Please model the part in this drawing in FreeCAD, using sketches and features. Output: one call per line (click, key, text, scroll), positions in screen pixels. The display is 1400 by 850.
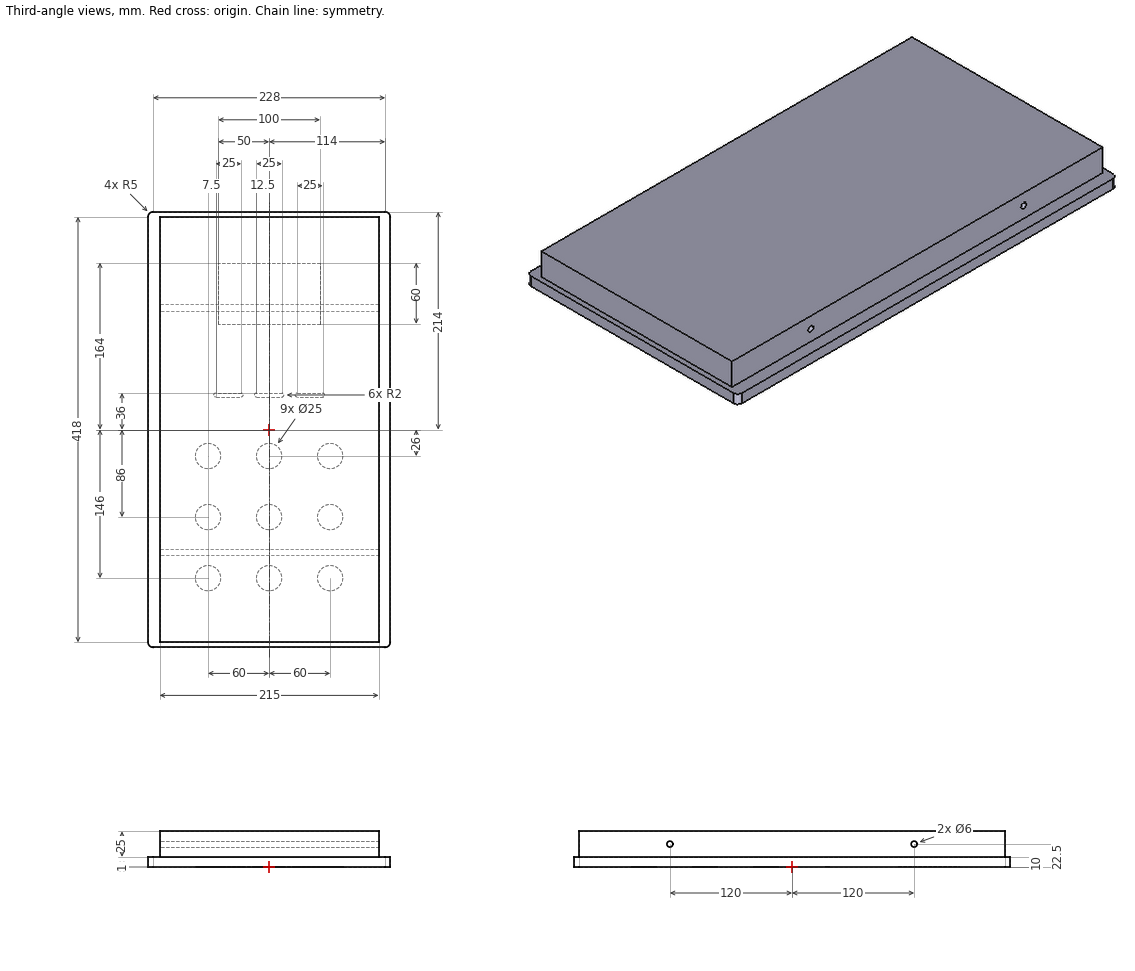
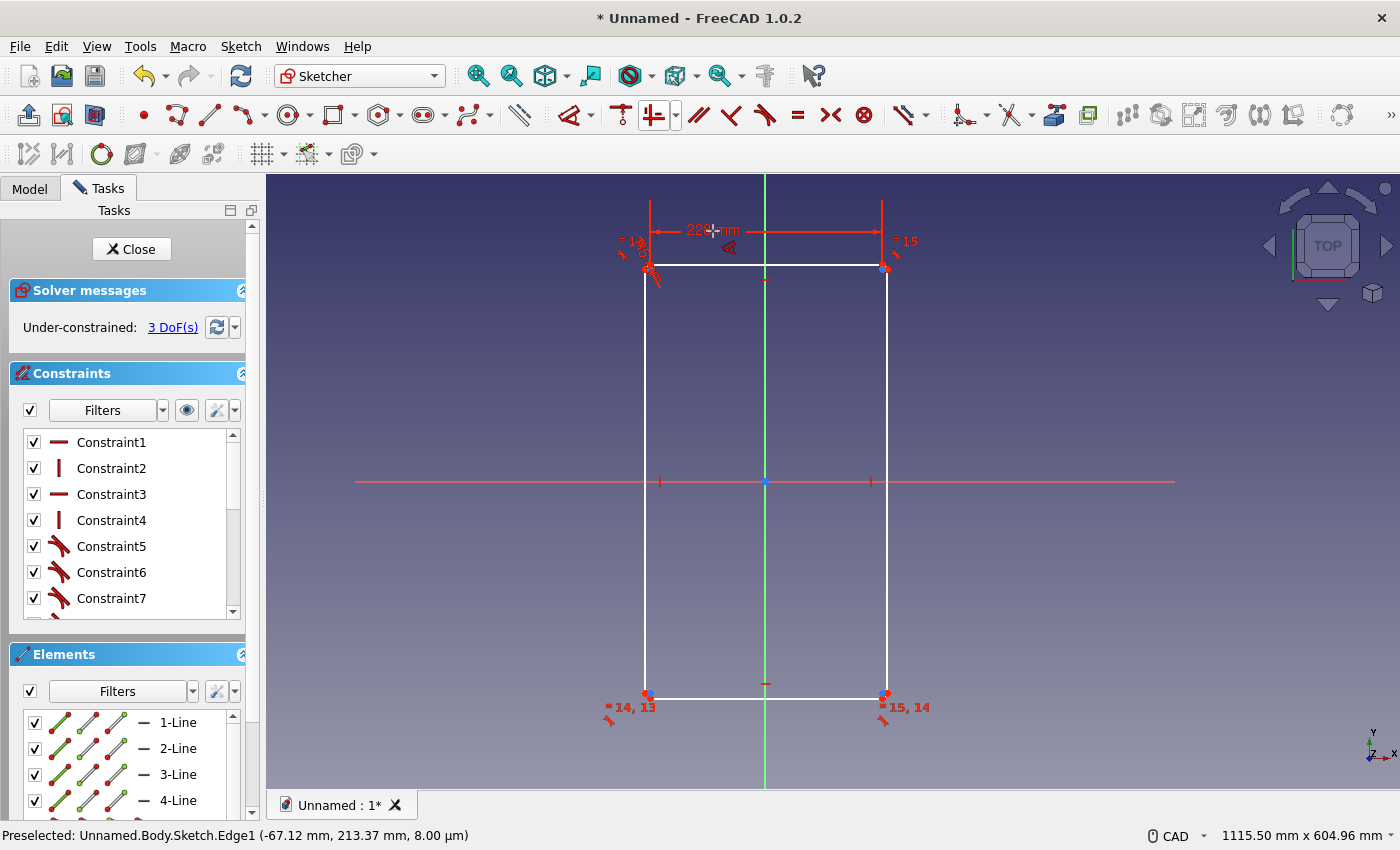
click(645, 397)
click(611, 384)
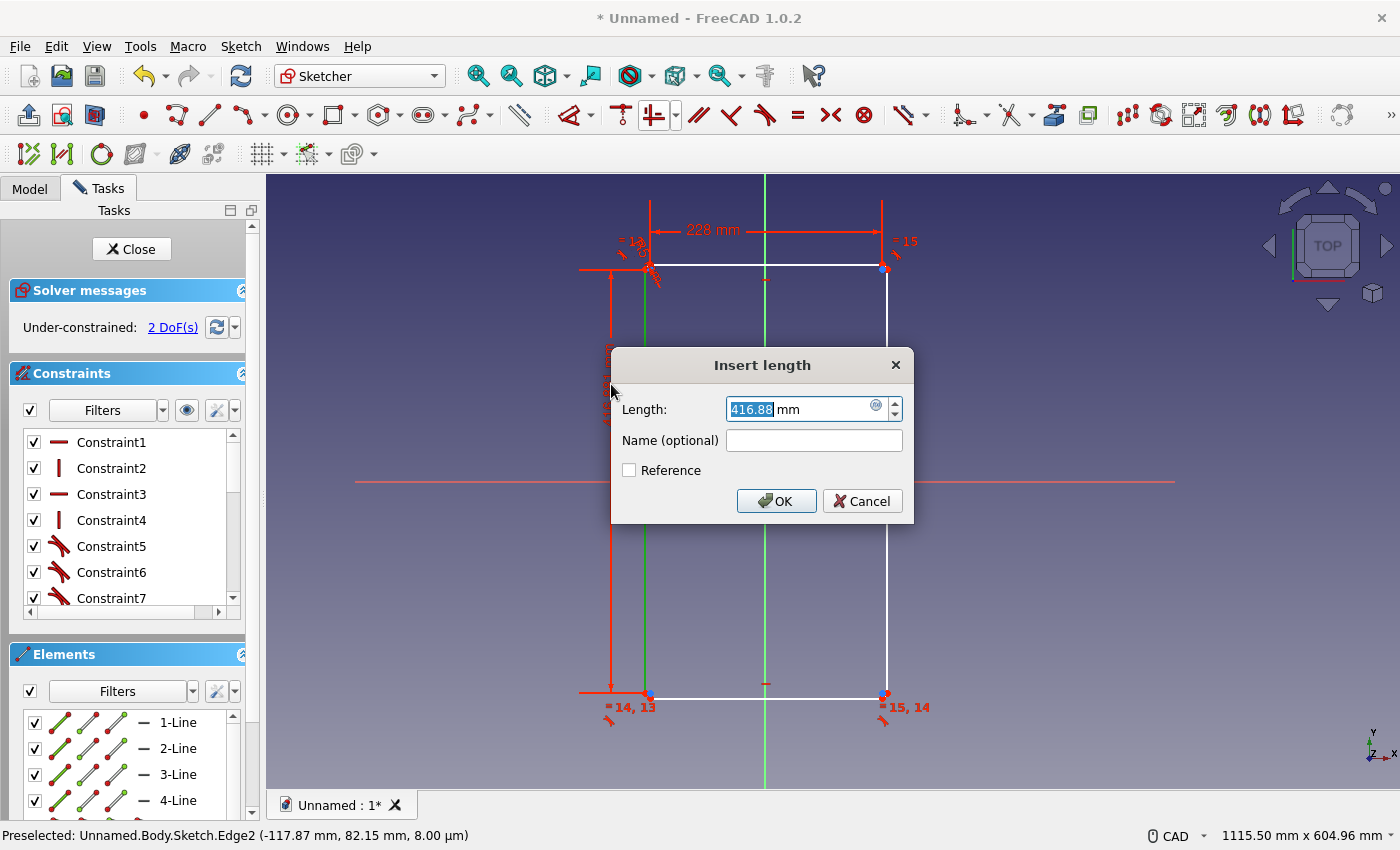
text(418)
key(Return)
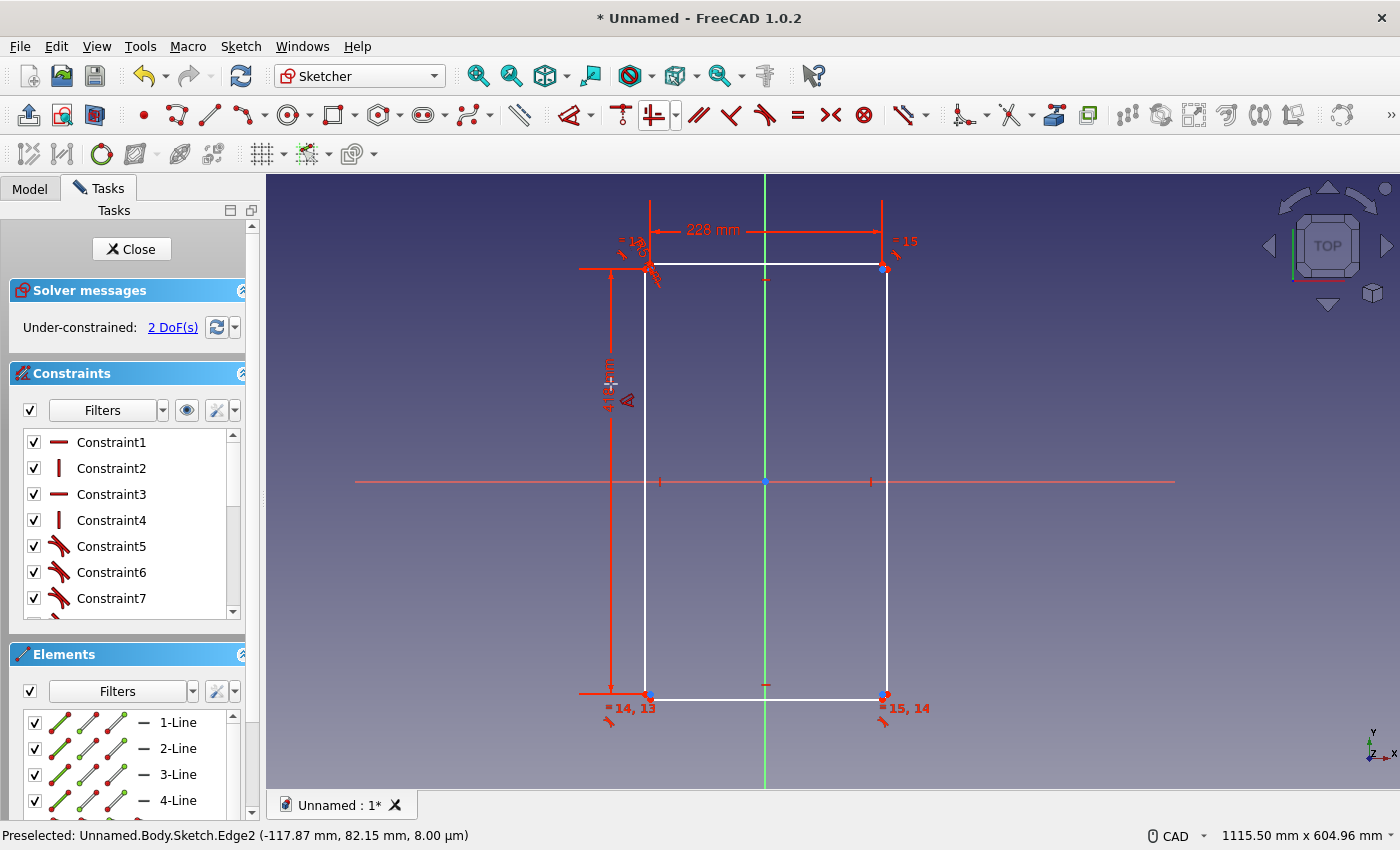
scroll(882, 264, up, 5)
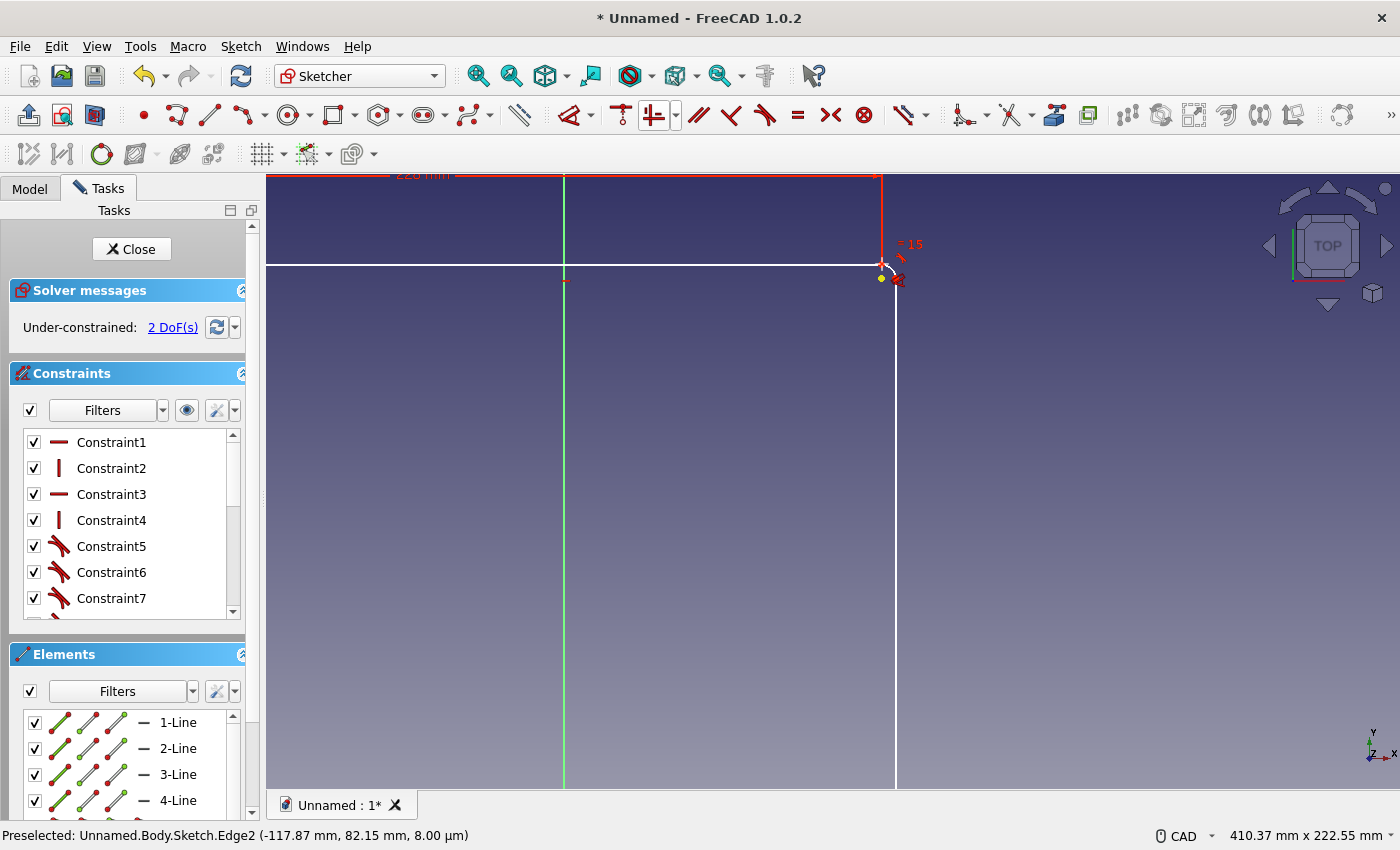
click(882, 265)
click(723, 231)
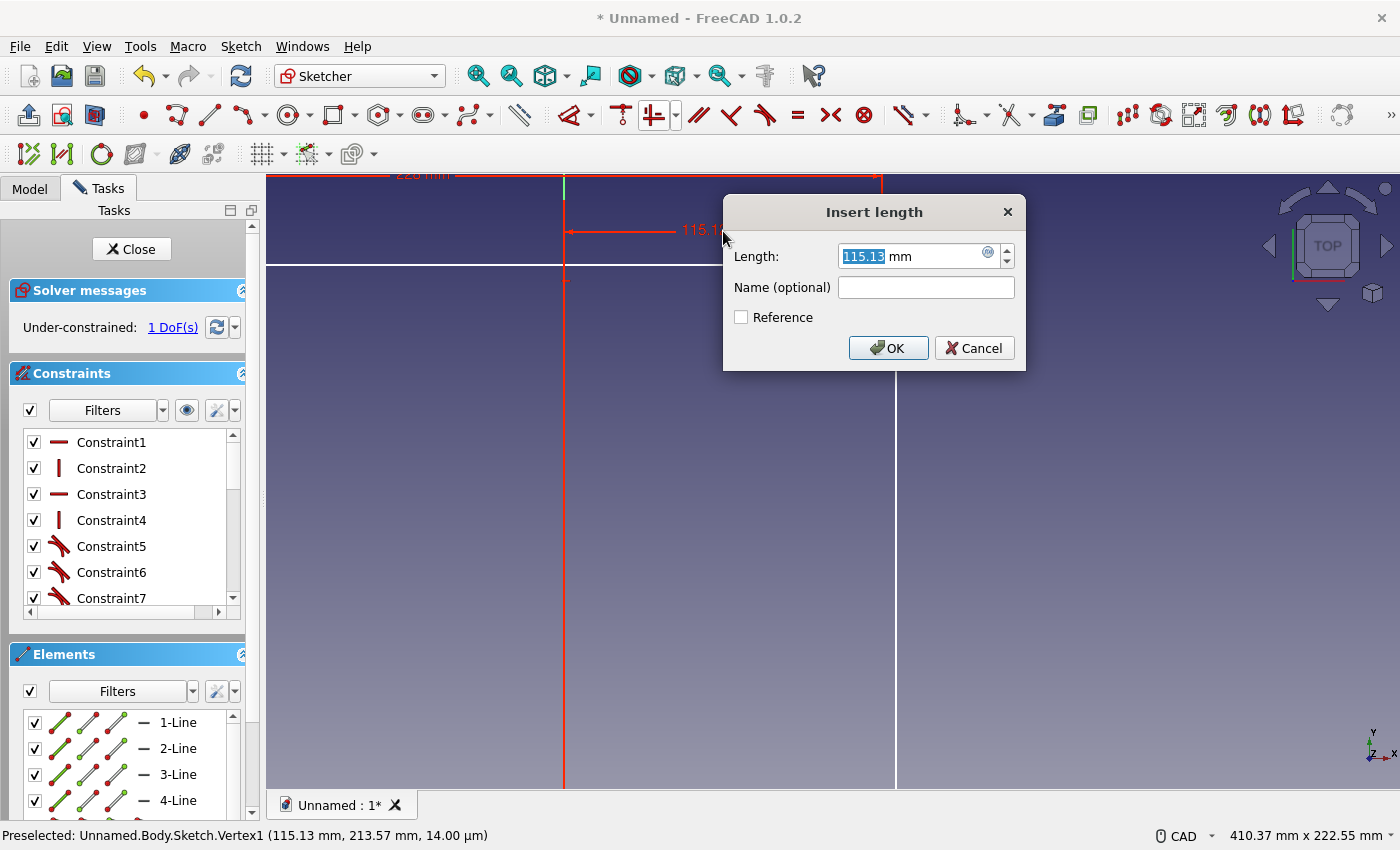
text(114)
key(Return)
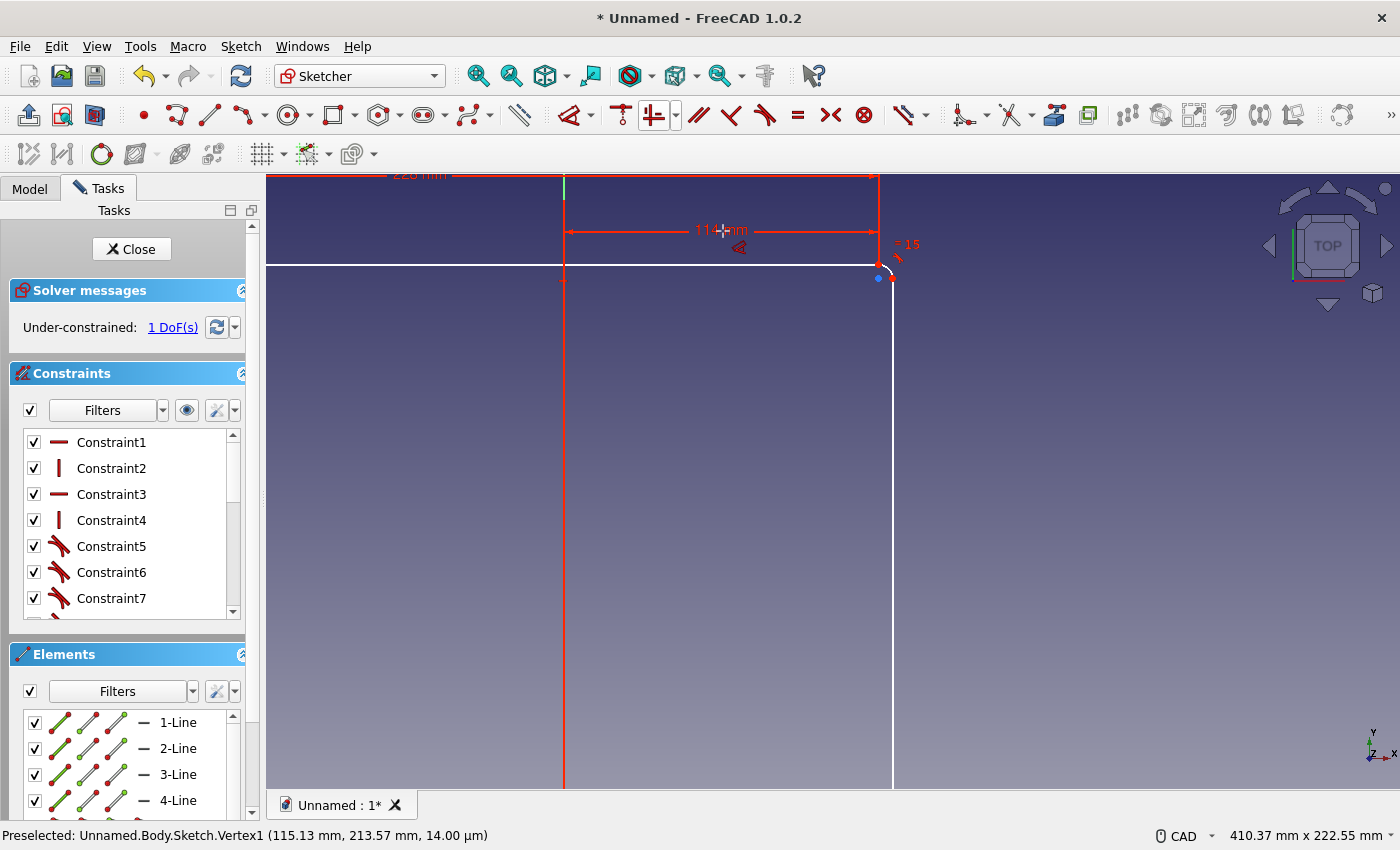
click(879, 265)
click(913, 513)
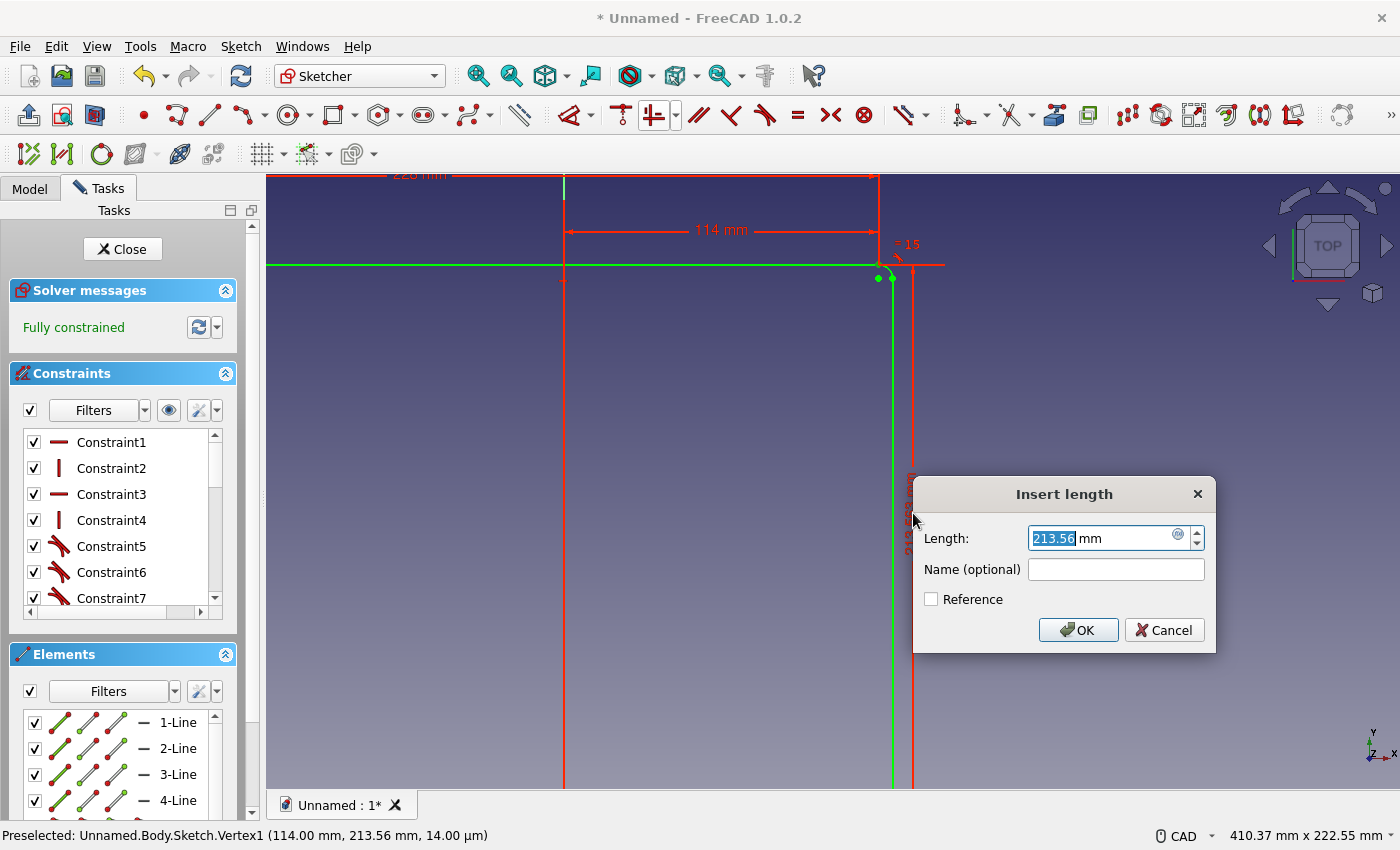
text(214)
key(Return)
key(Escape)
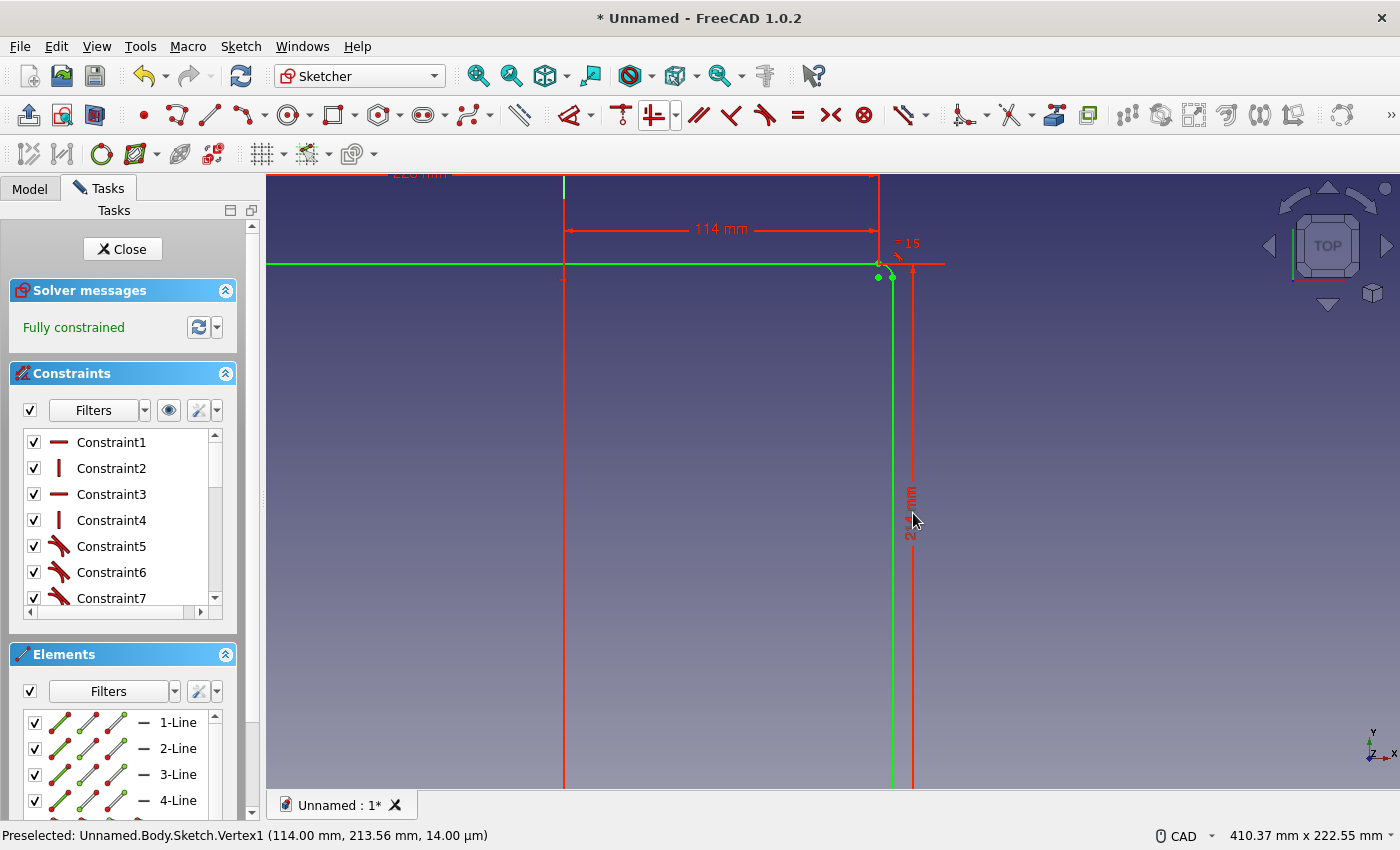
click(123, 249)